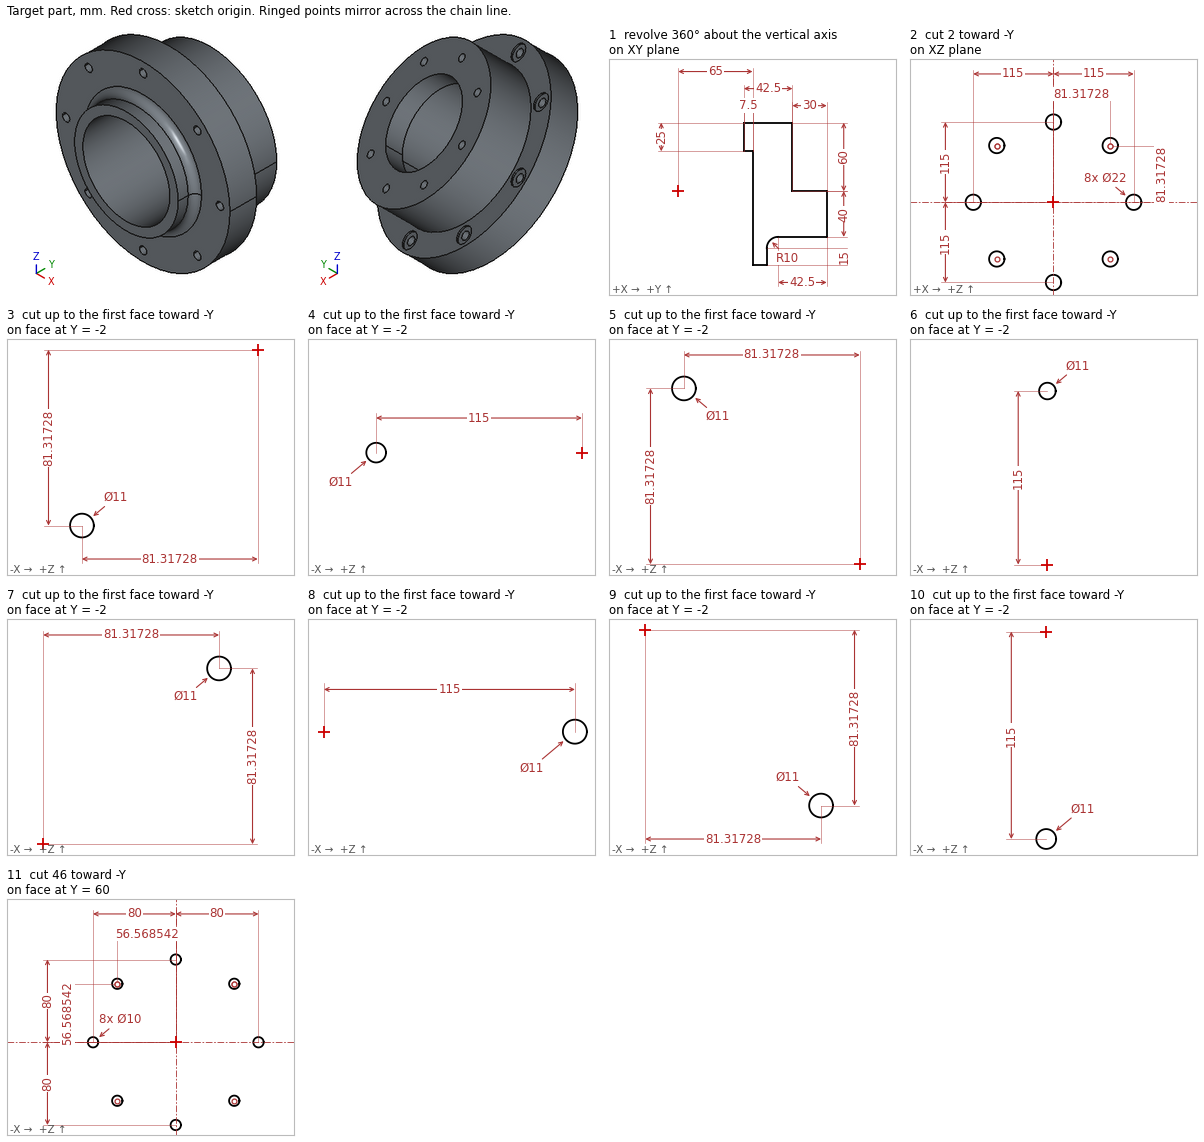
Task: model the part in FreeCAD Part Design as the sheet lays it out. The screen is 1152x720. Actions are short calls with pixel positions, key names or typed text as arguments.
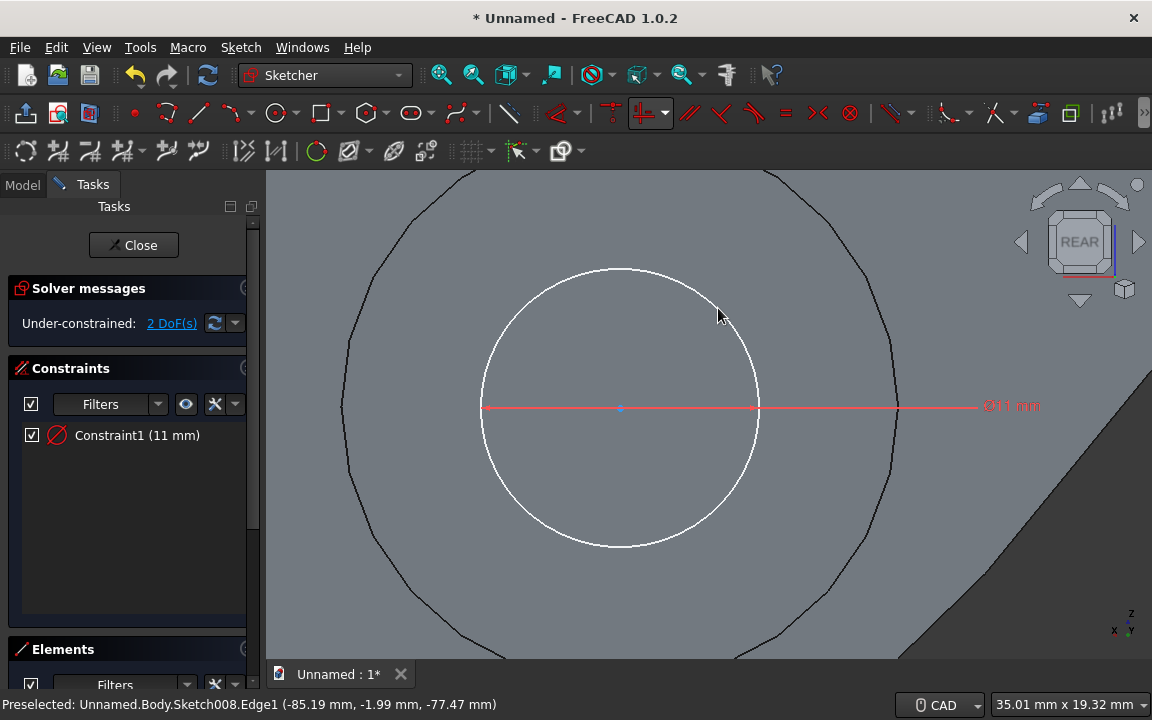
click(556, 114)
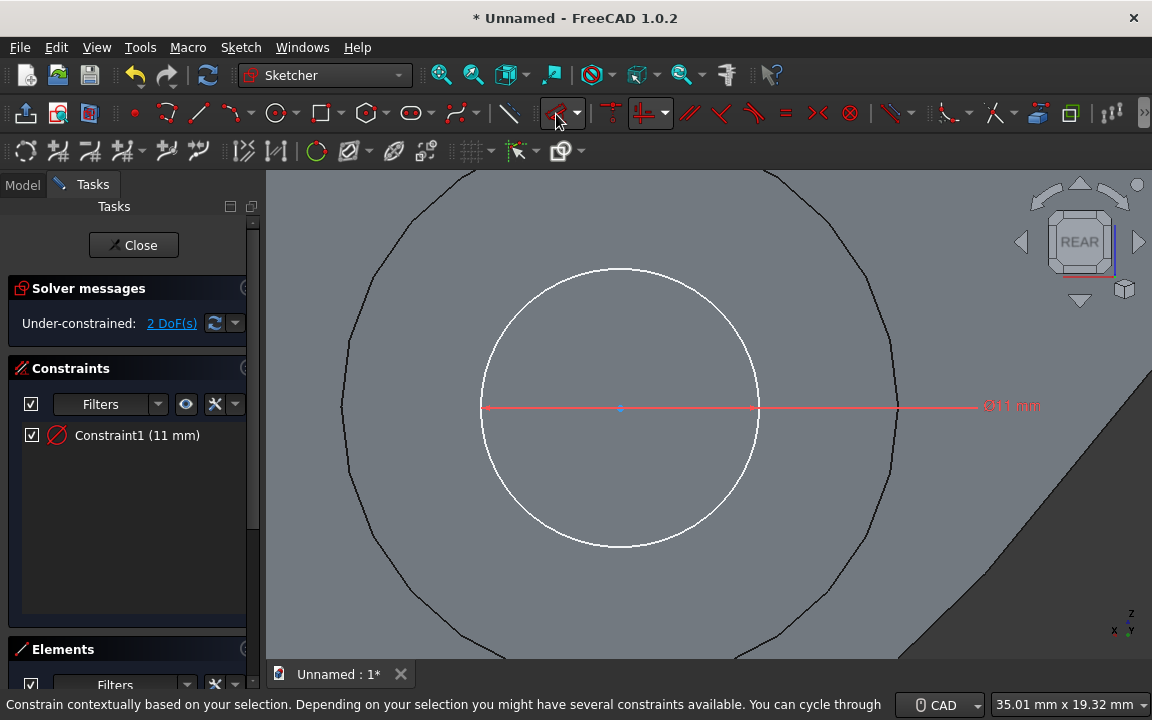
click(620, 408)
click(457, 442)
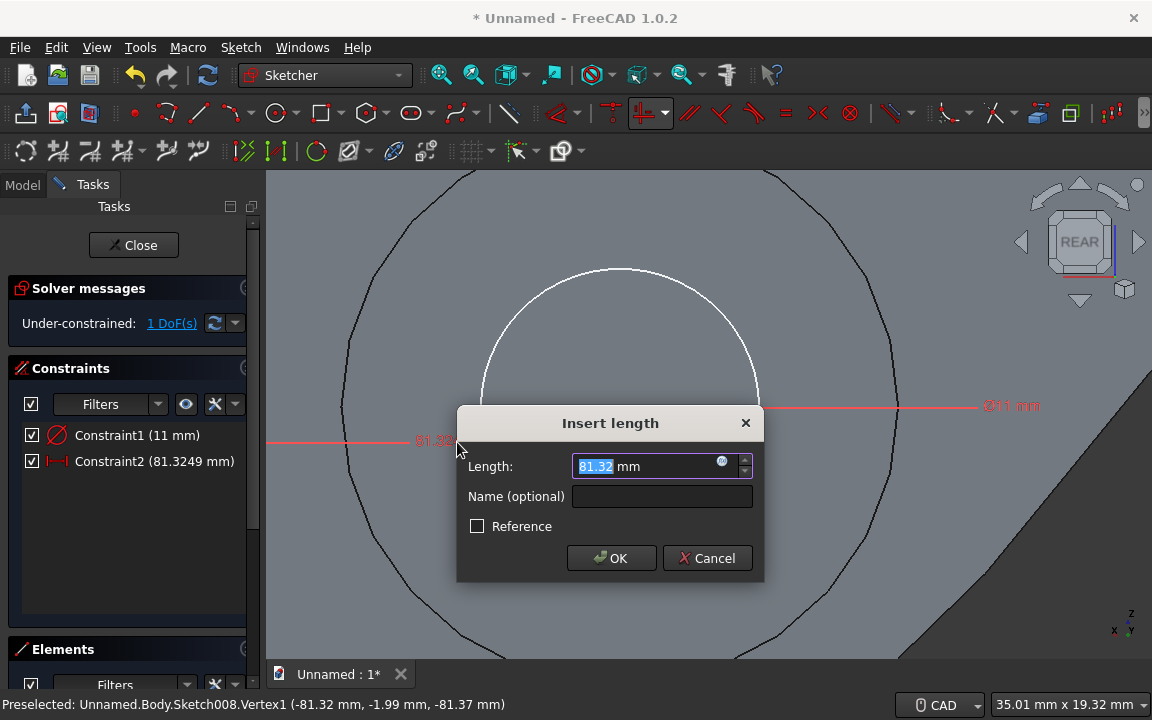
text(81.31728)
key(Return)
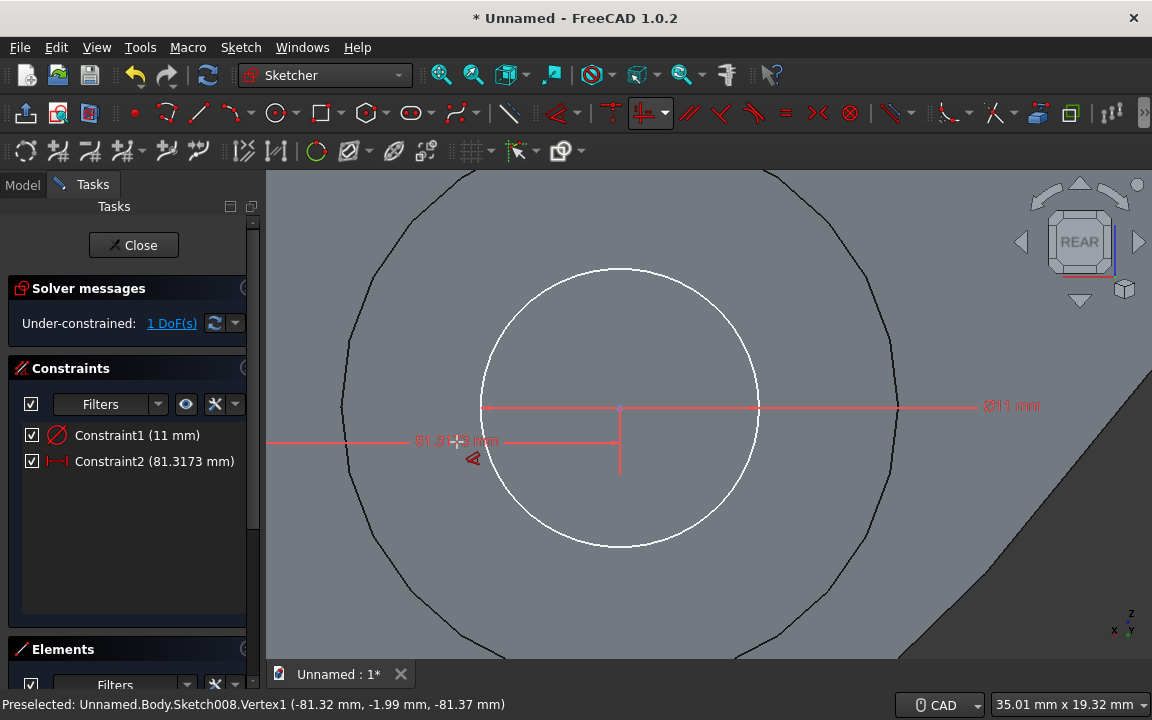
click(620, 408)
click(654, 303)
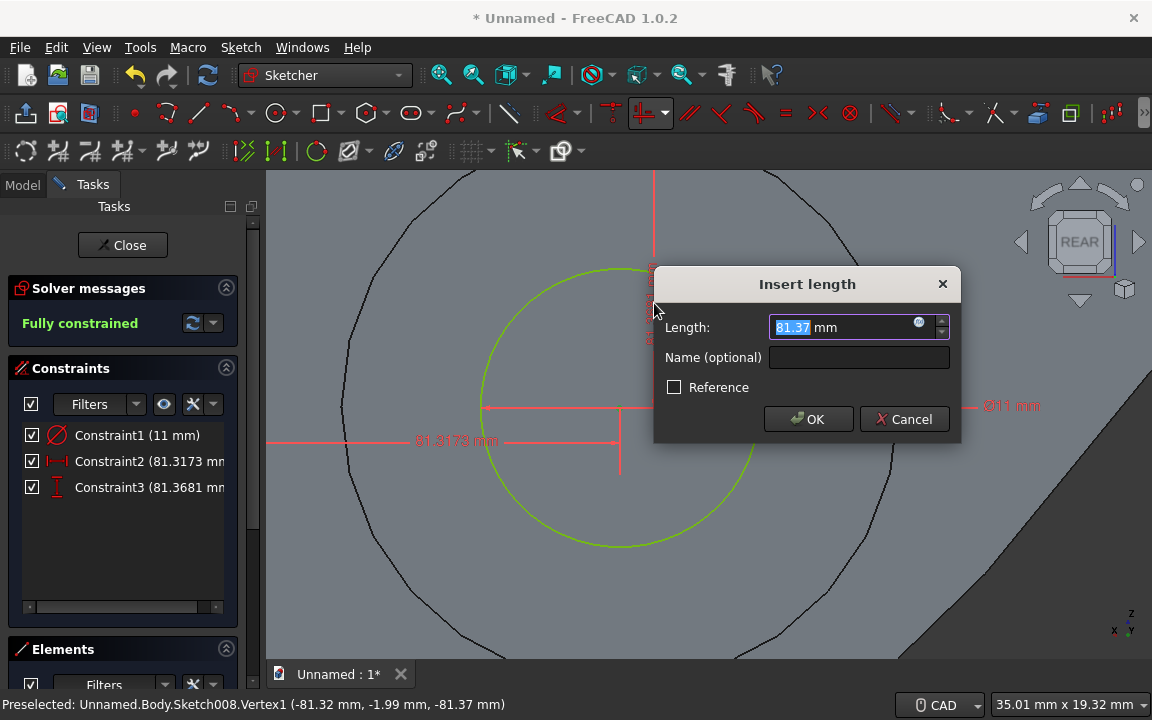
text(81.31728)
key(Return)
key(Escape)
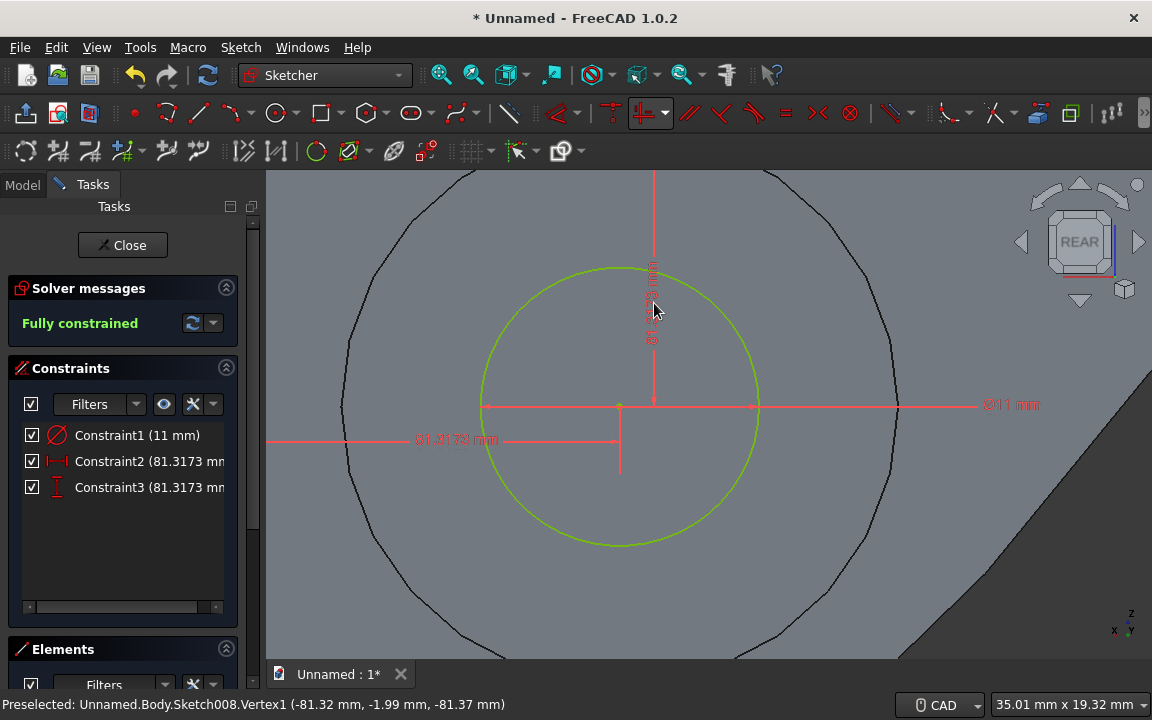
click(123, 245)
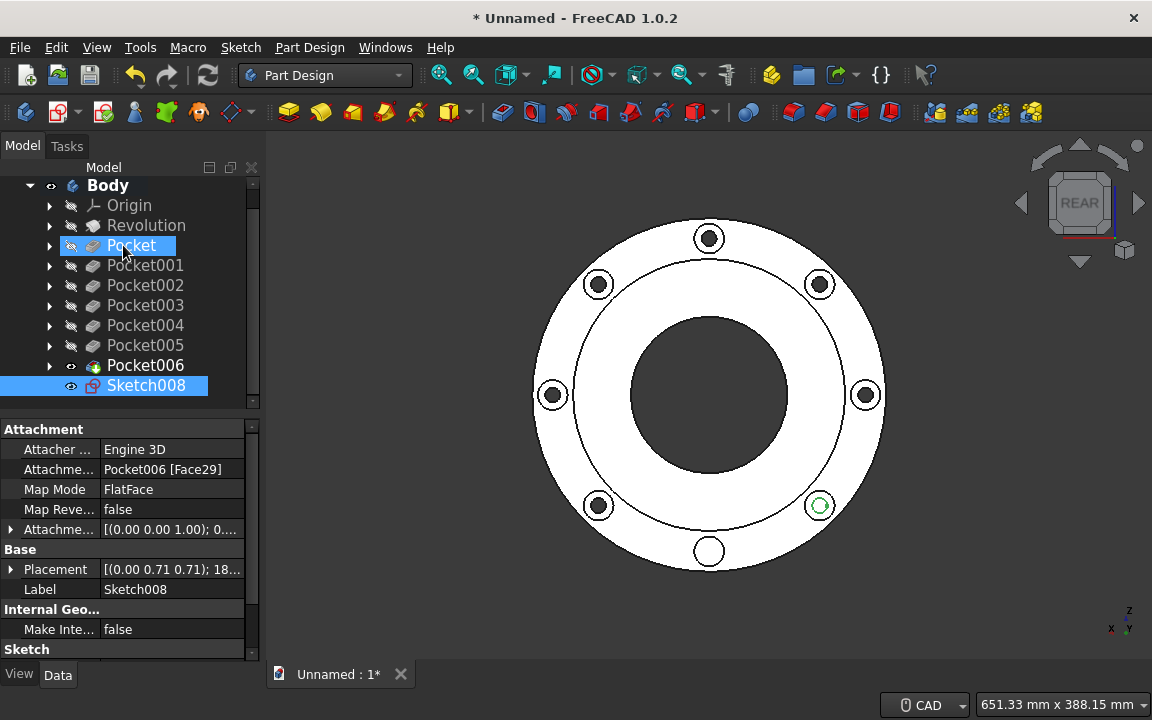
click(504, 112)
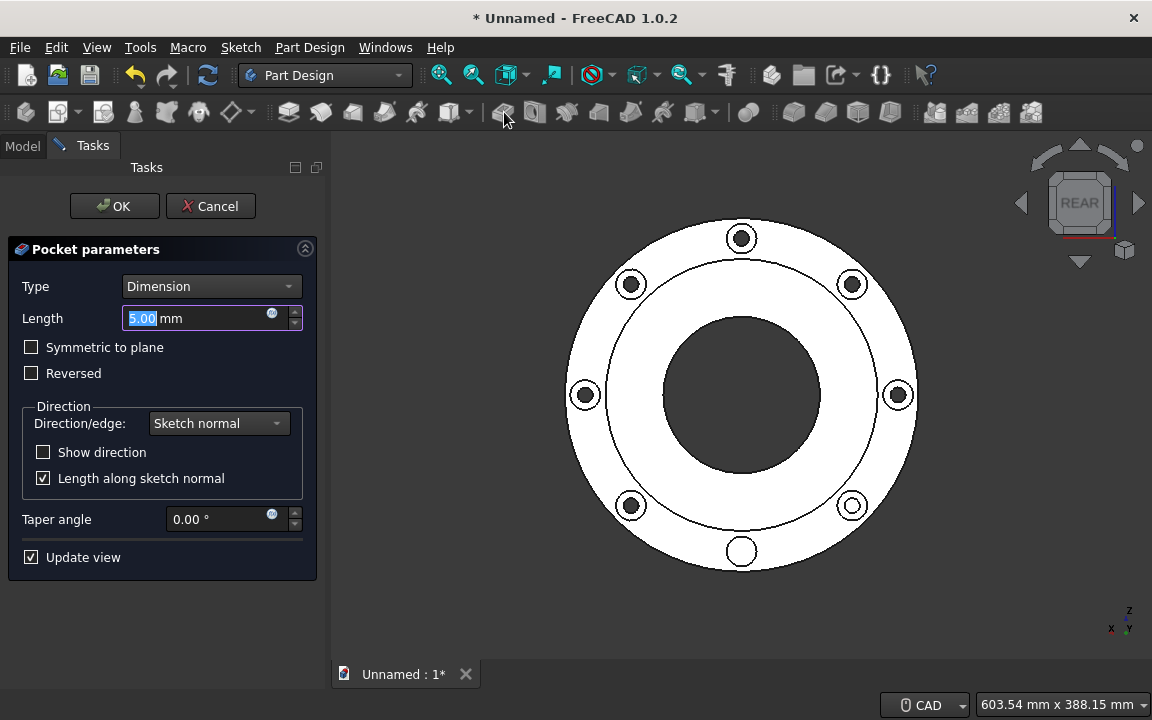
click(212, 286)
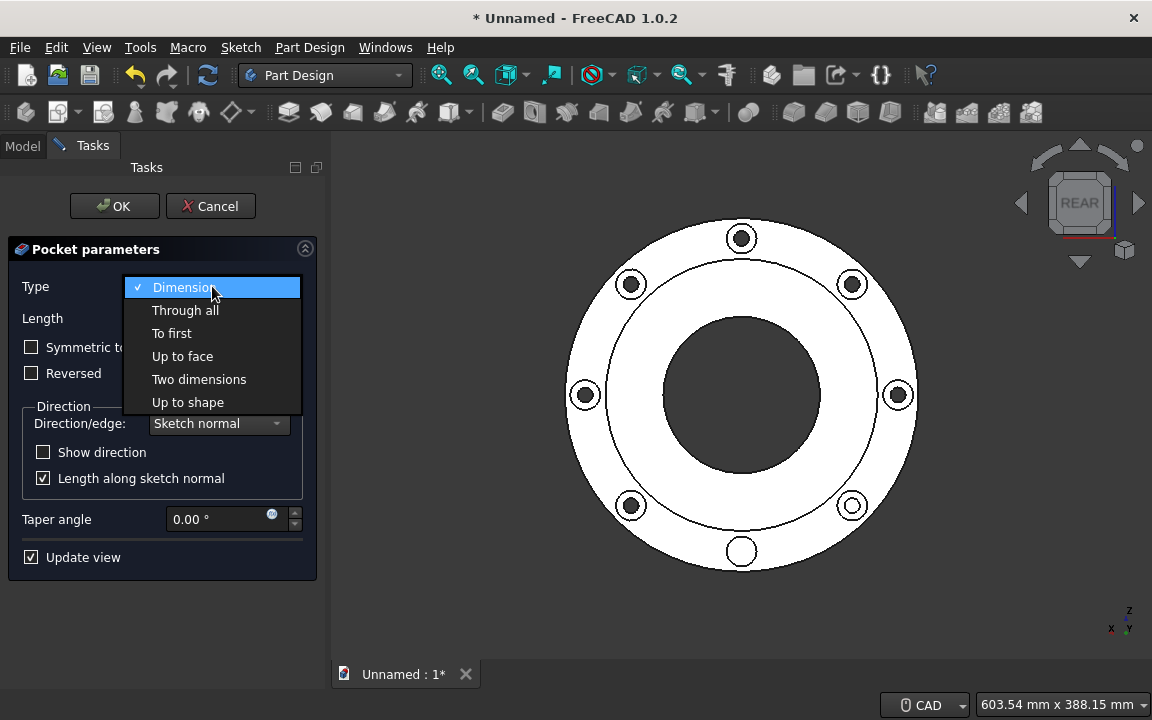
click(212, 334)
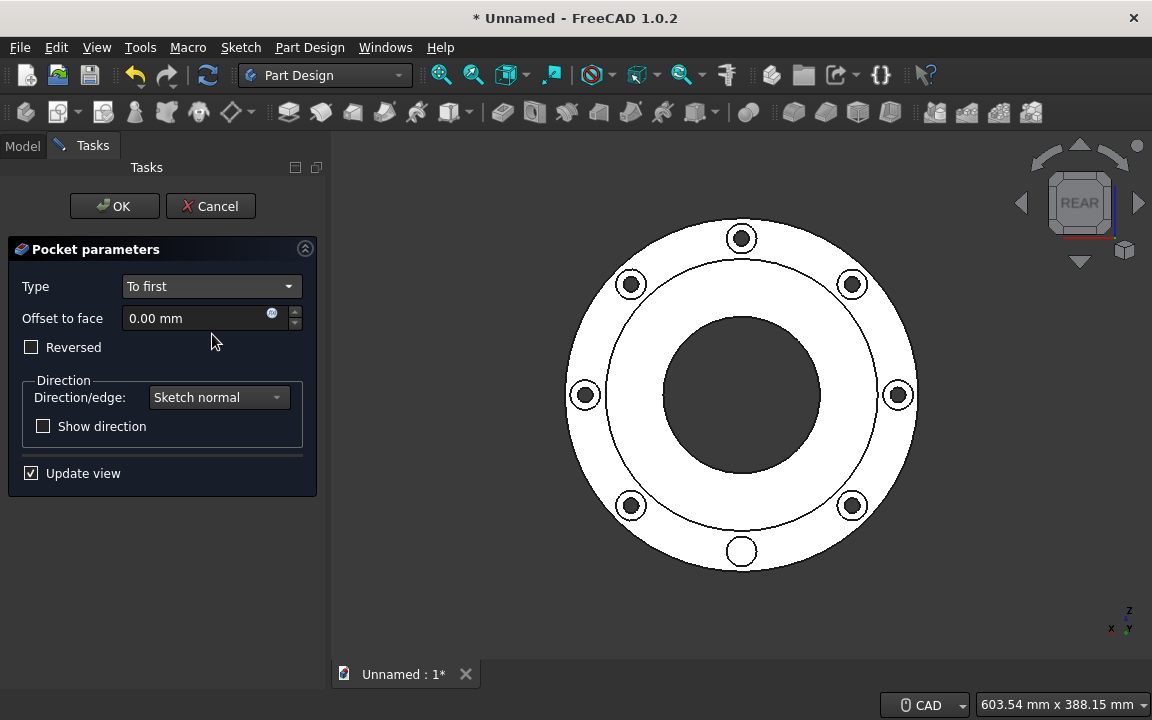
click(115, 206)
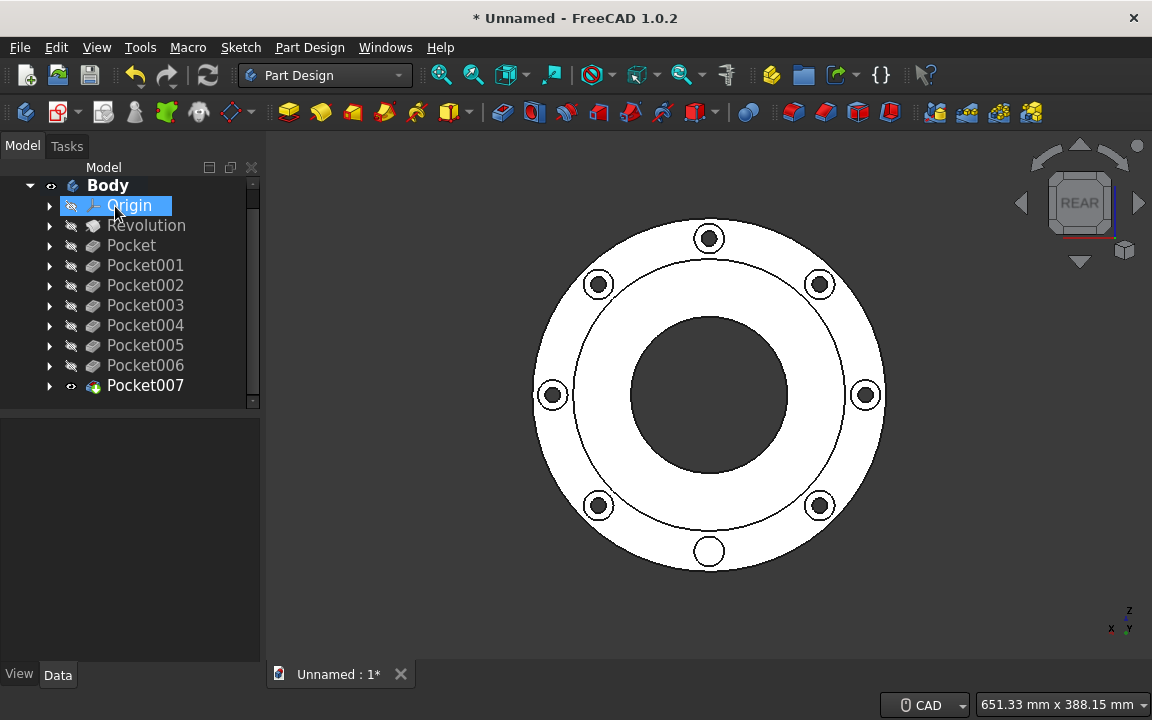
click(709, 550)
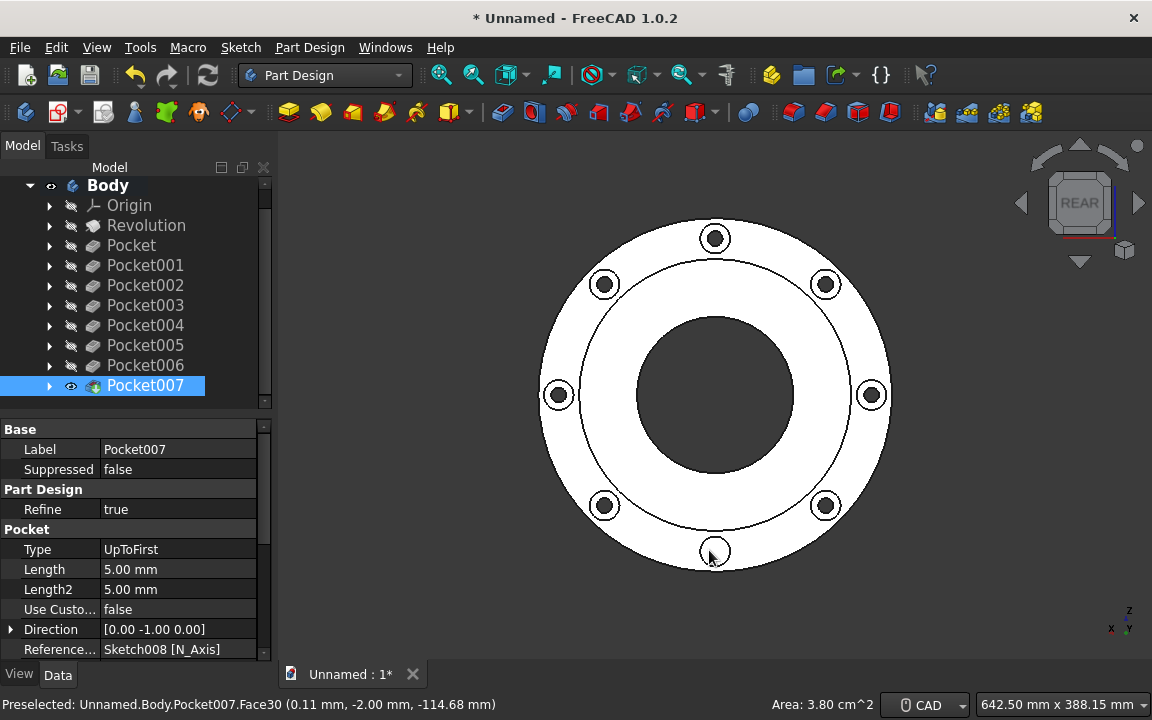
click(58, 112)